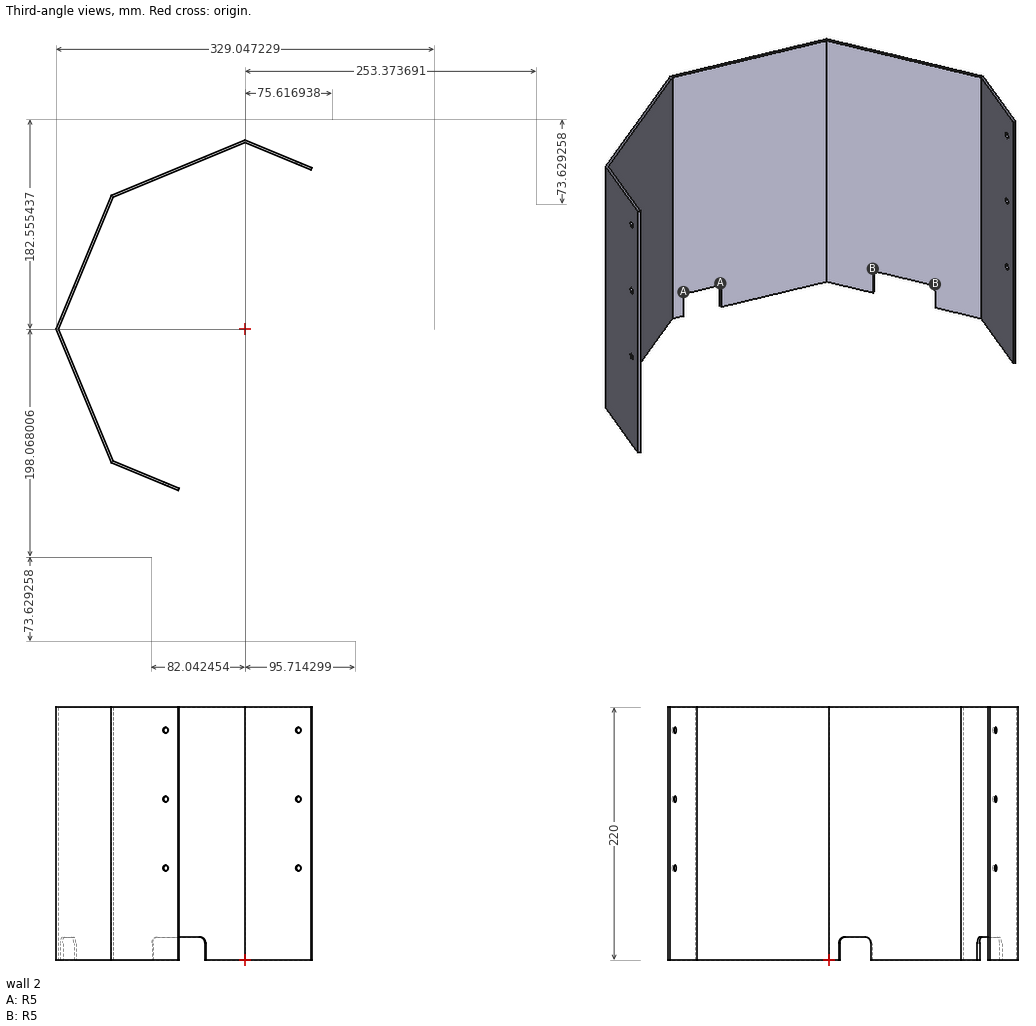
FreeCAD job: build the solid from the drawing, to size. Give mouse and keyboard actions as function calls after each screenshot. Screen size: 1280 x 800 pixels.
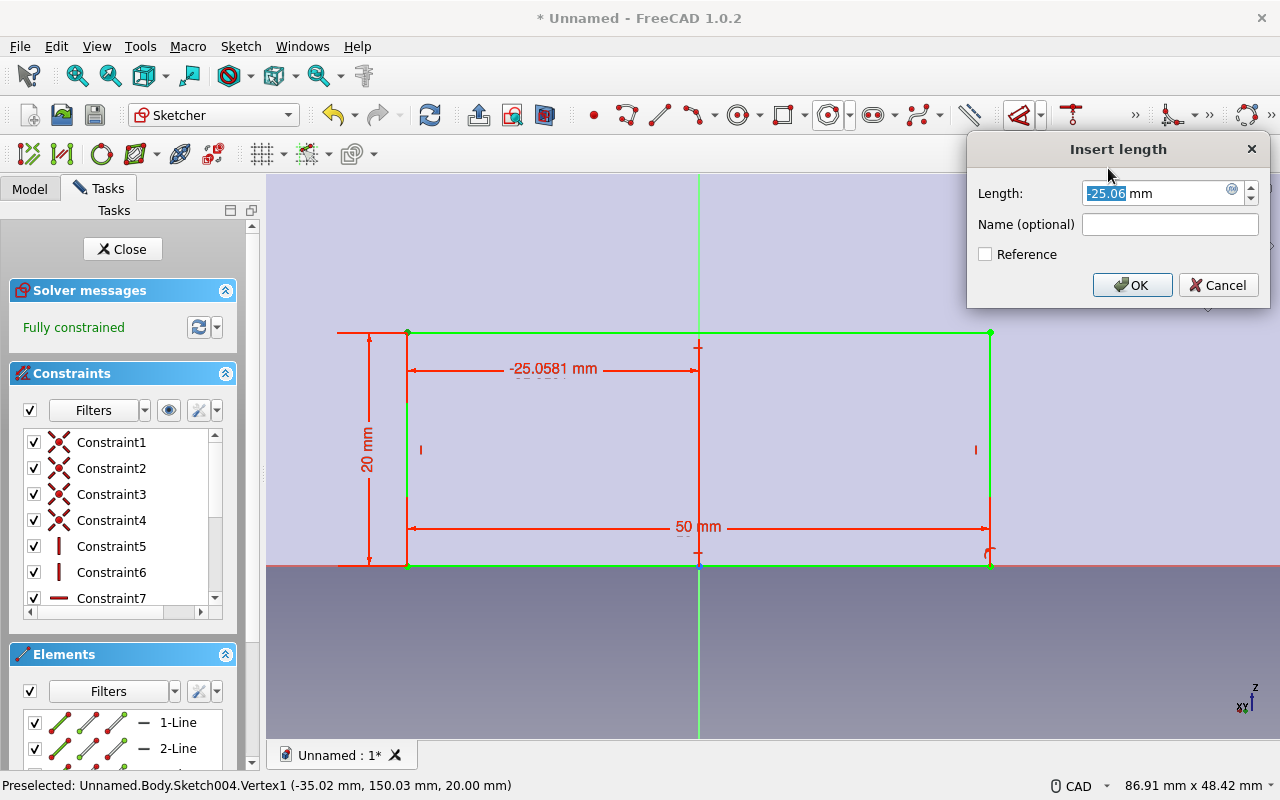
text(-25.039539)
key(Return)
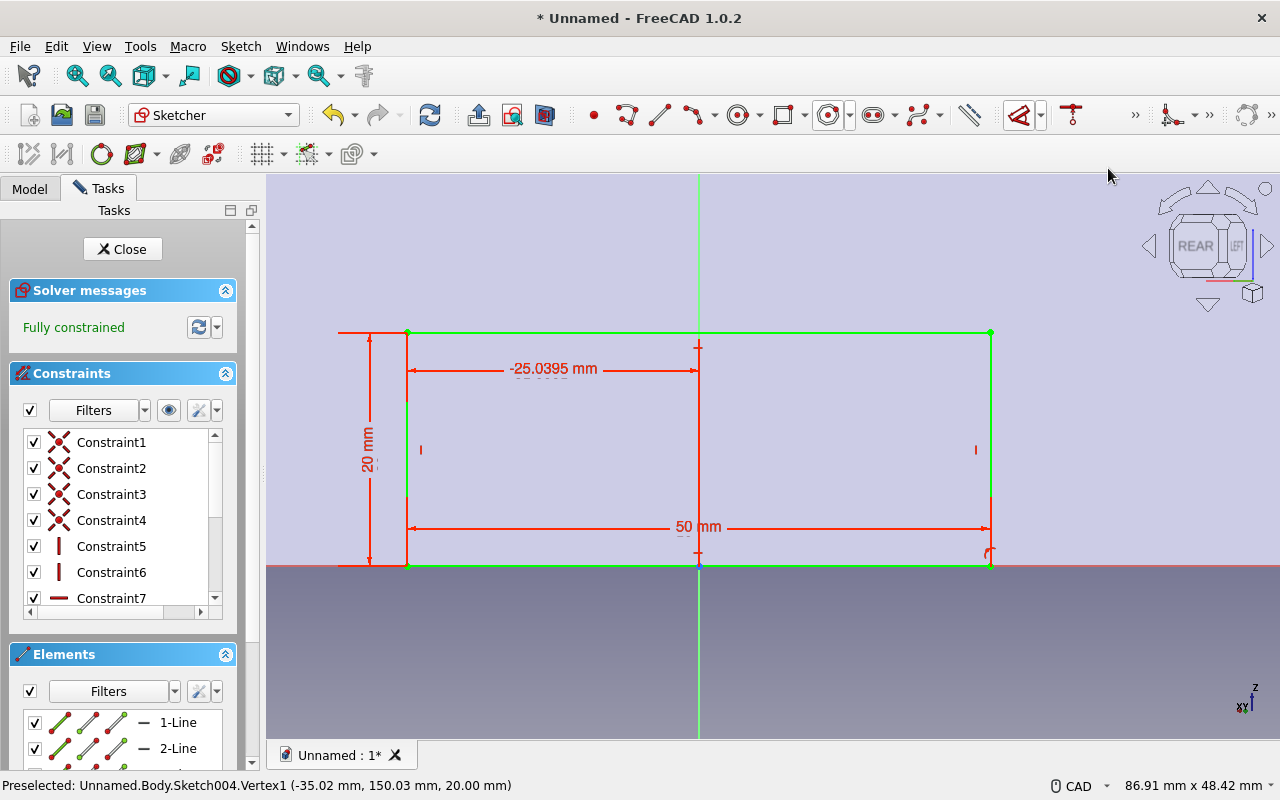
click(123, 249)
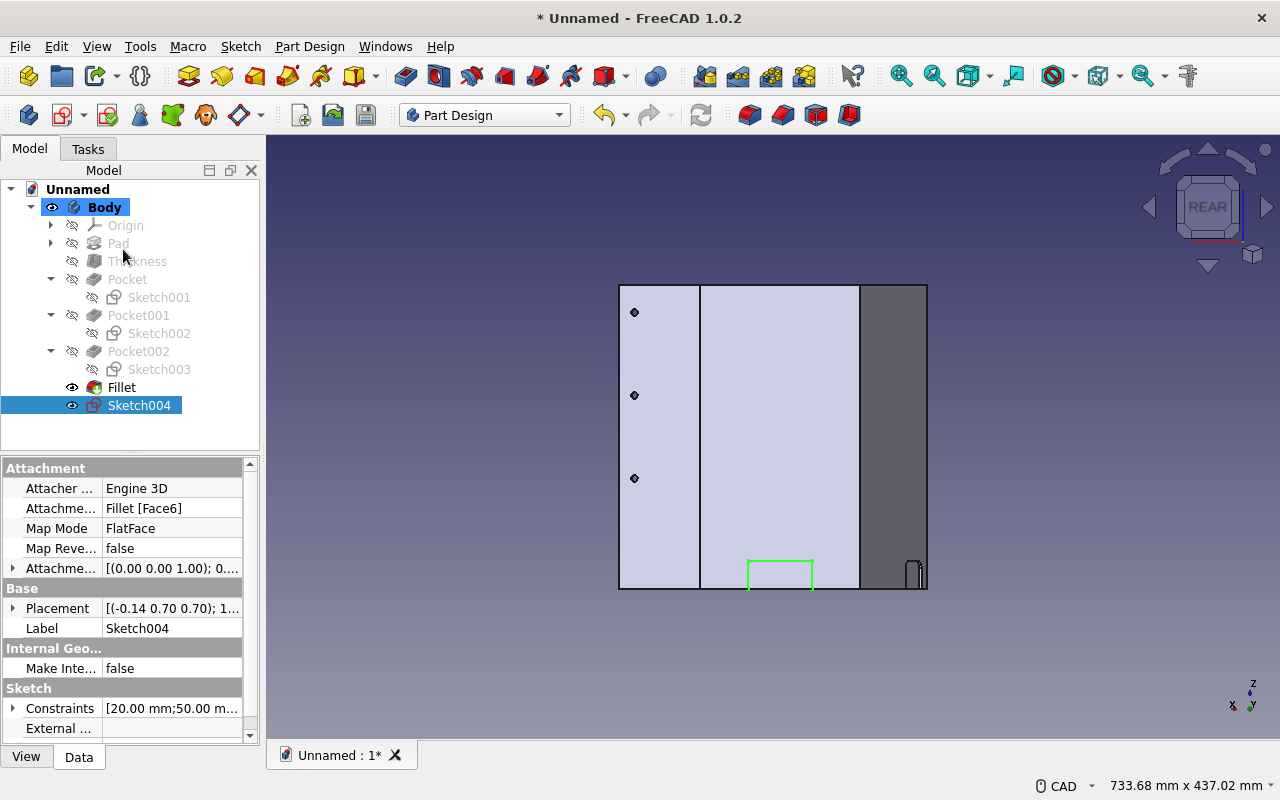
click(406, 76)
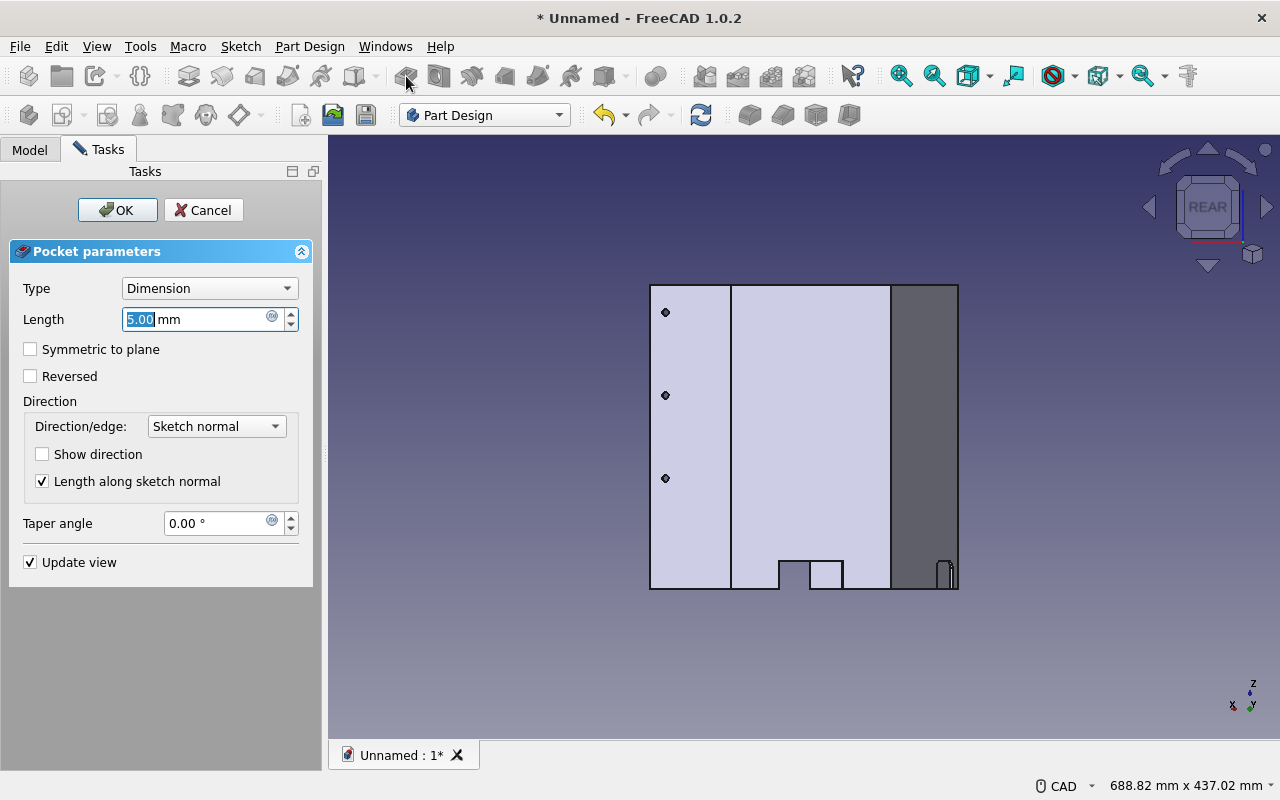
click(210, 288)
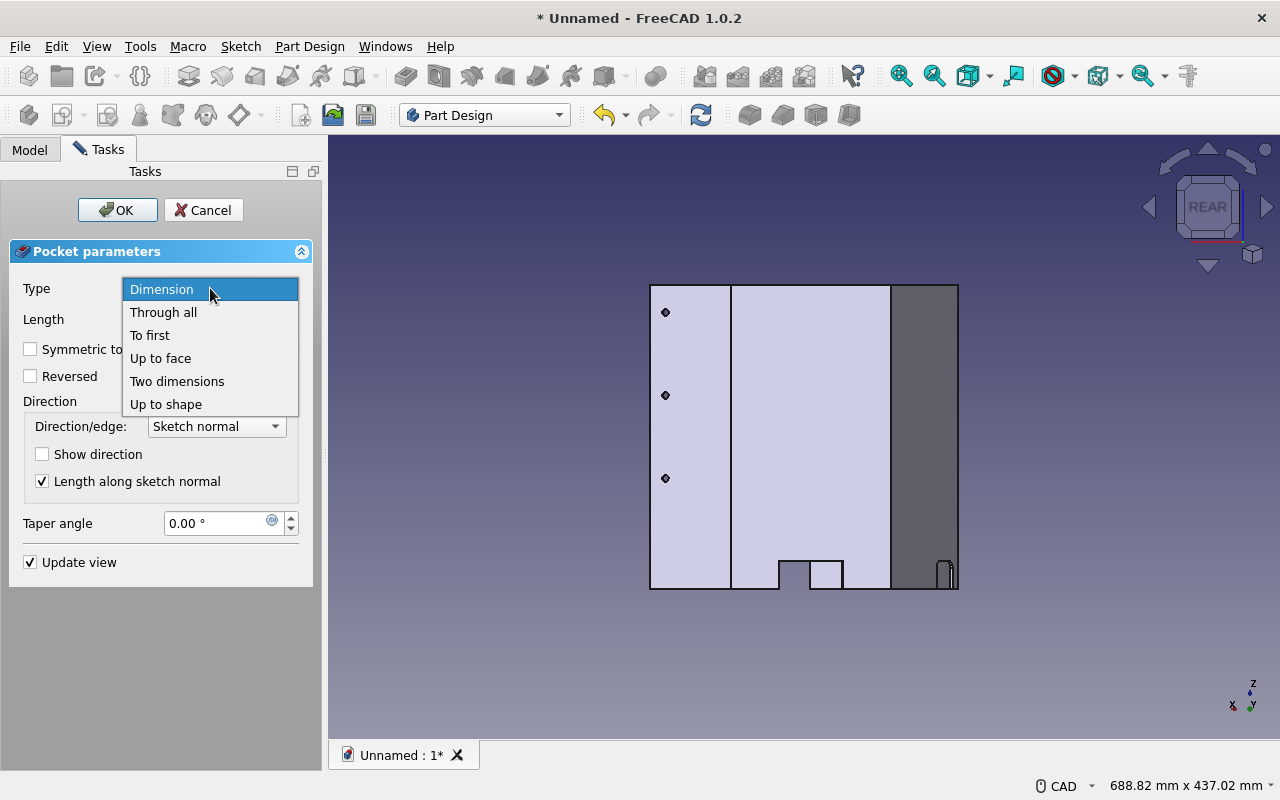
click(208, 312)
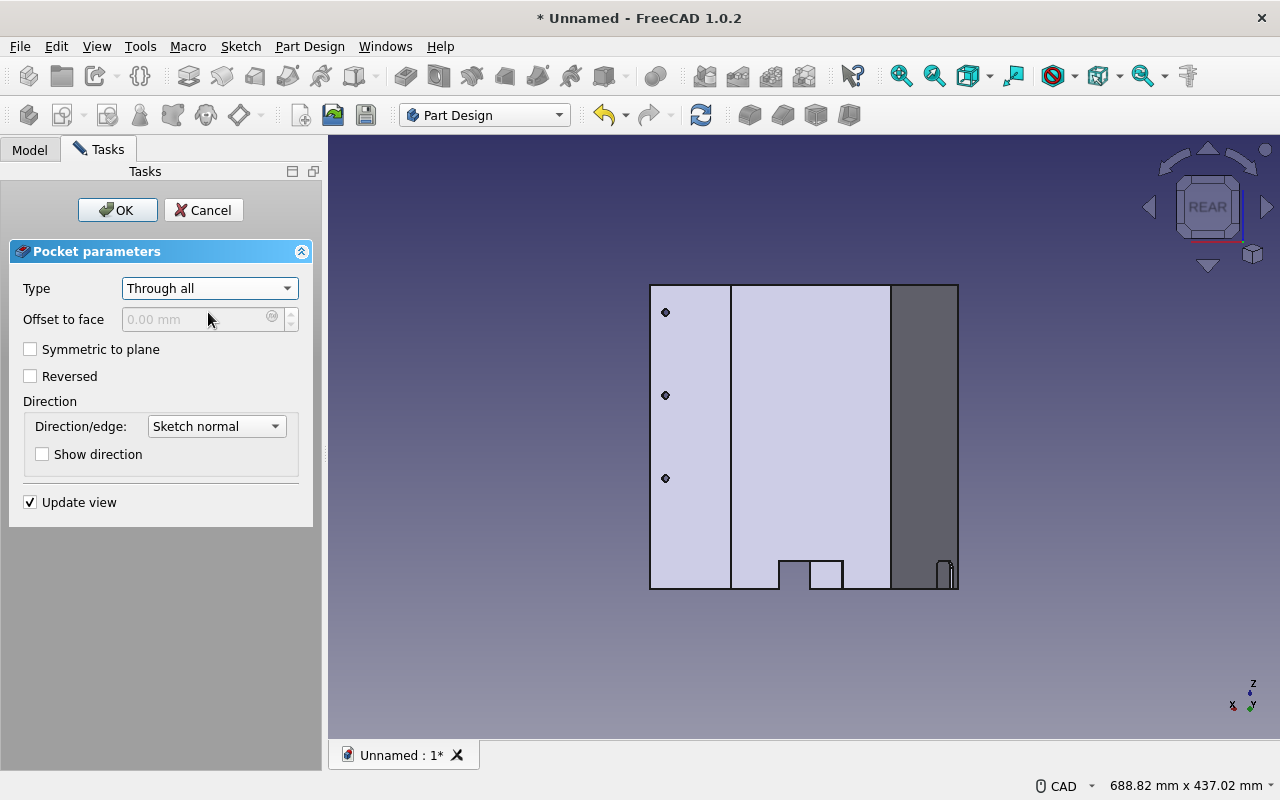
click(118, 210)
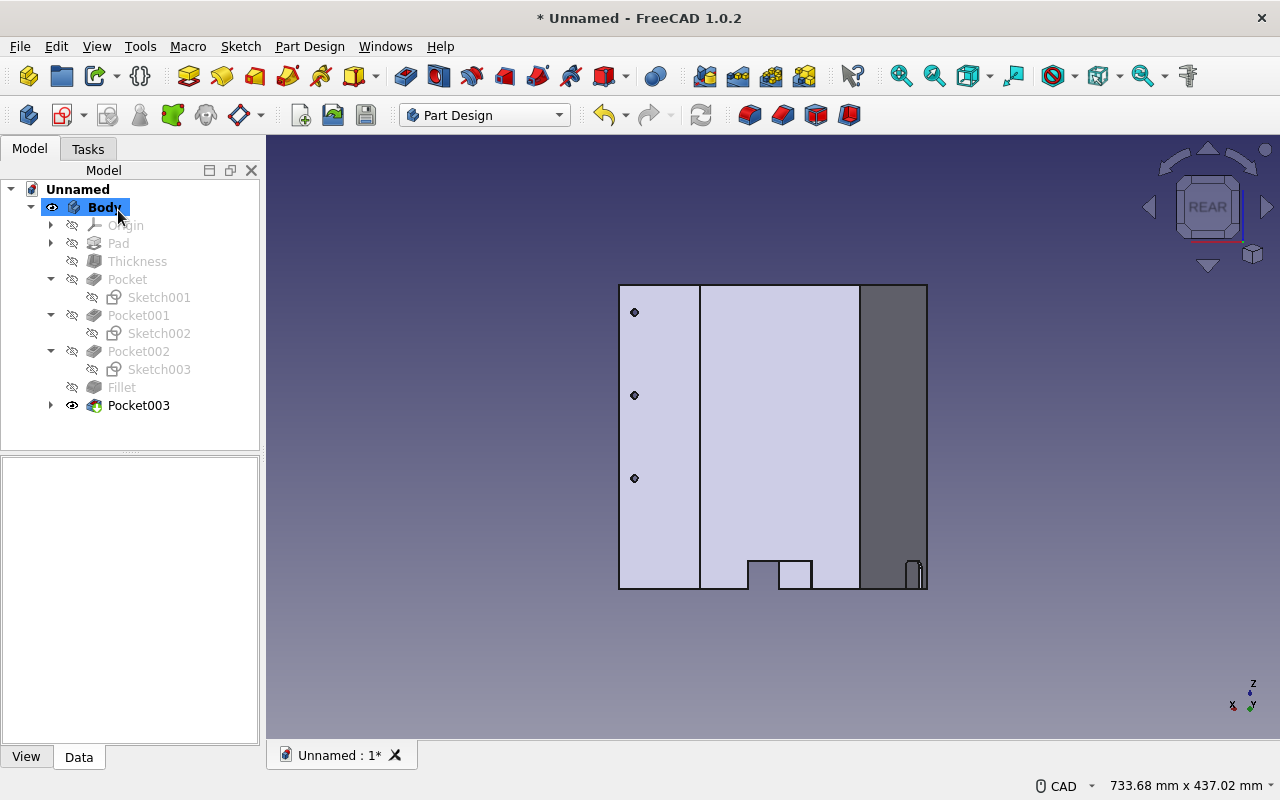
scroll(747, 560, up, 14)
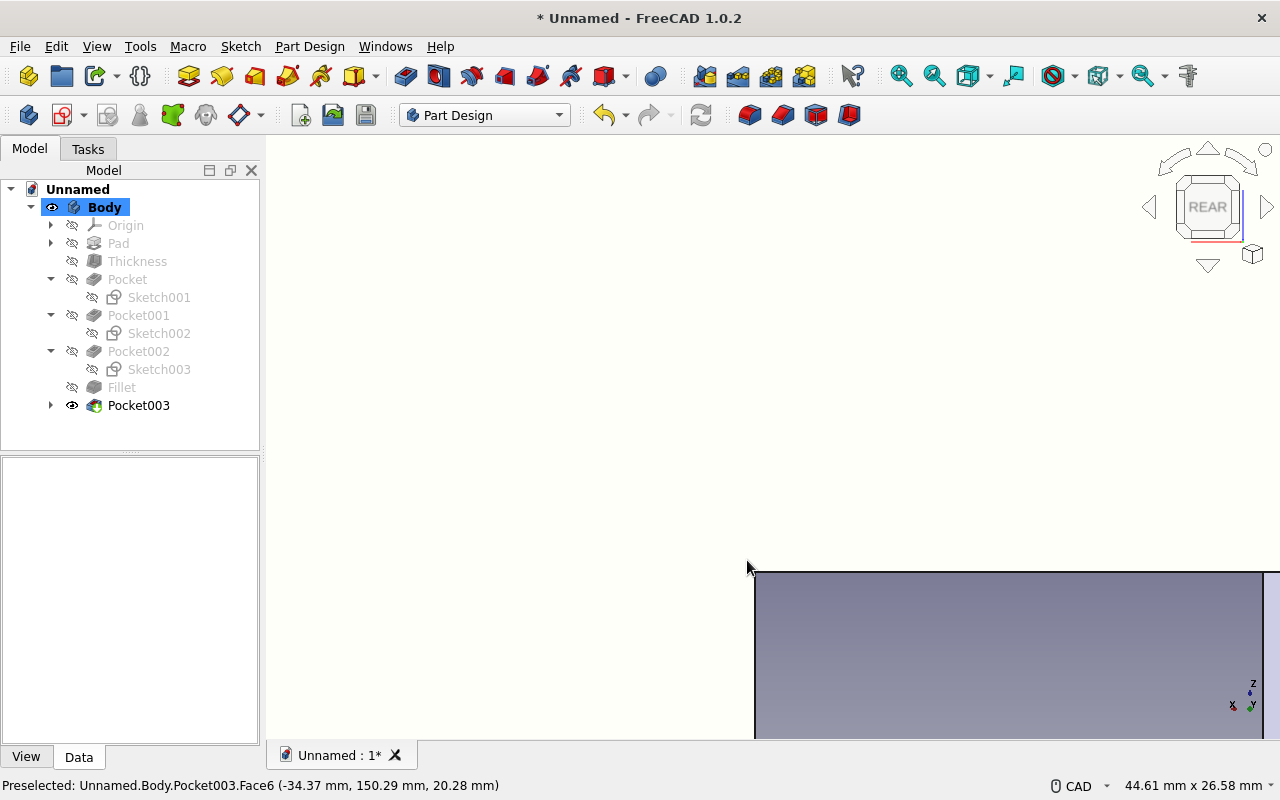
click(902, 76)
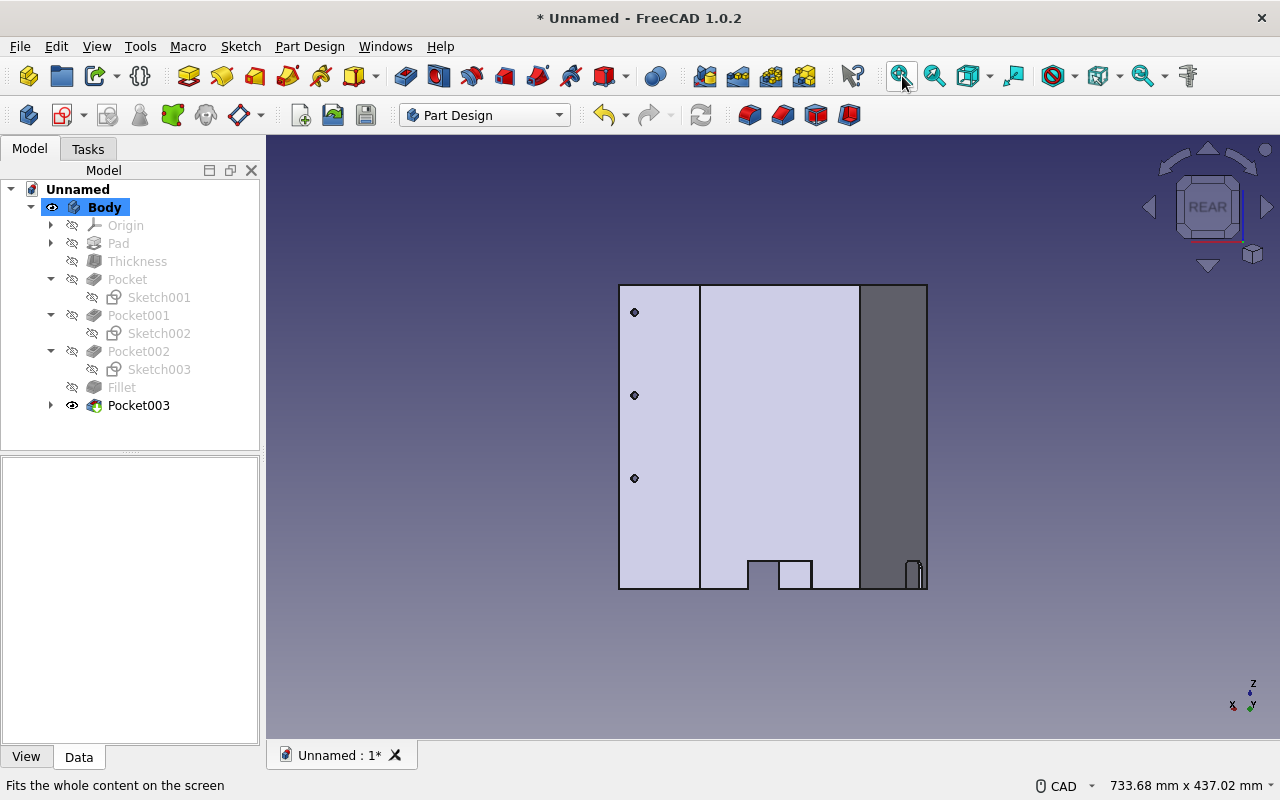
key(0)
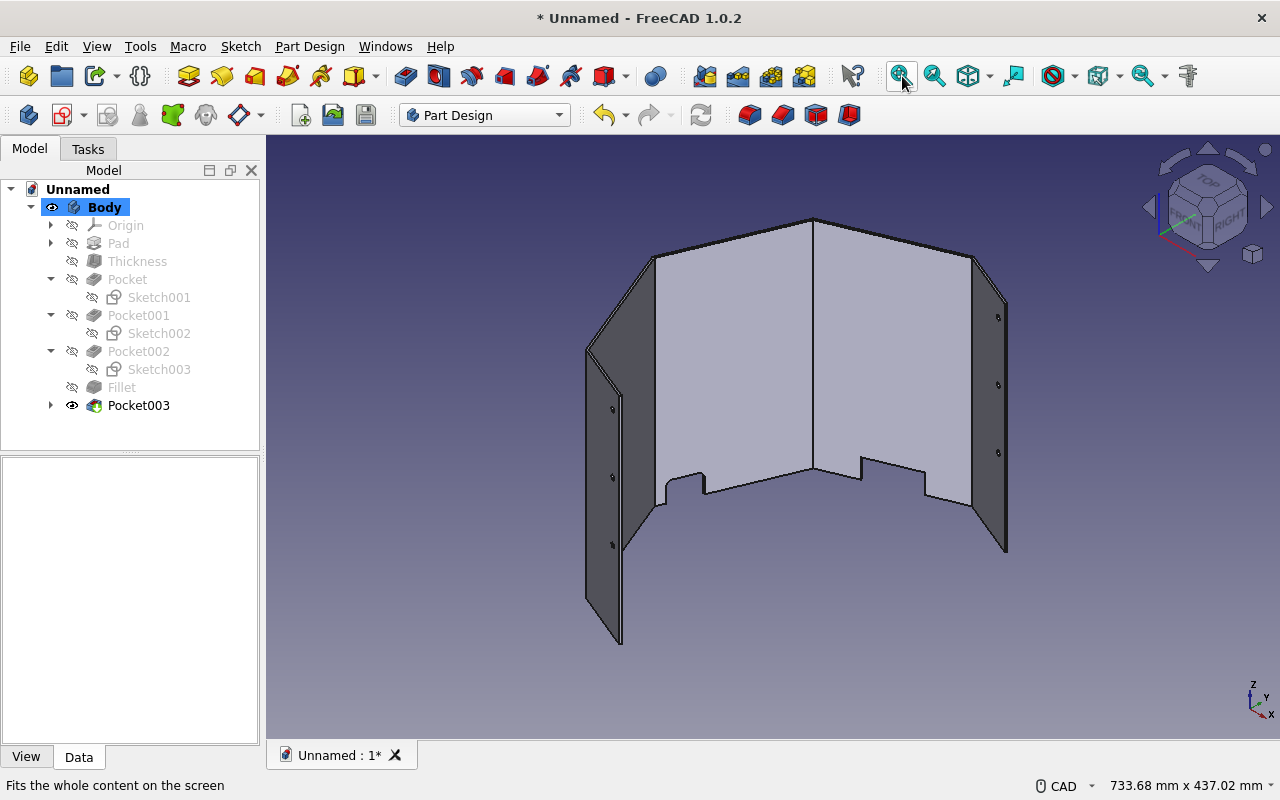
scroll(925, 471, up, 14)